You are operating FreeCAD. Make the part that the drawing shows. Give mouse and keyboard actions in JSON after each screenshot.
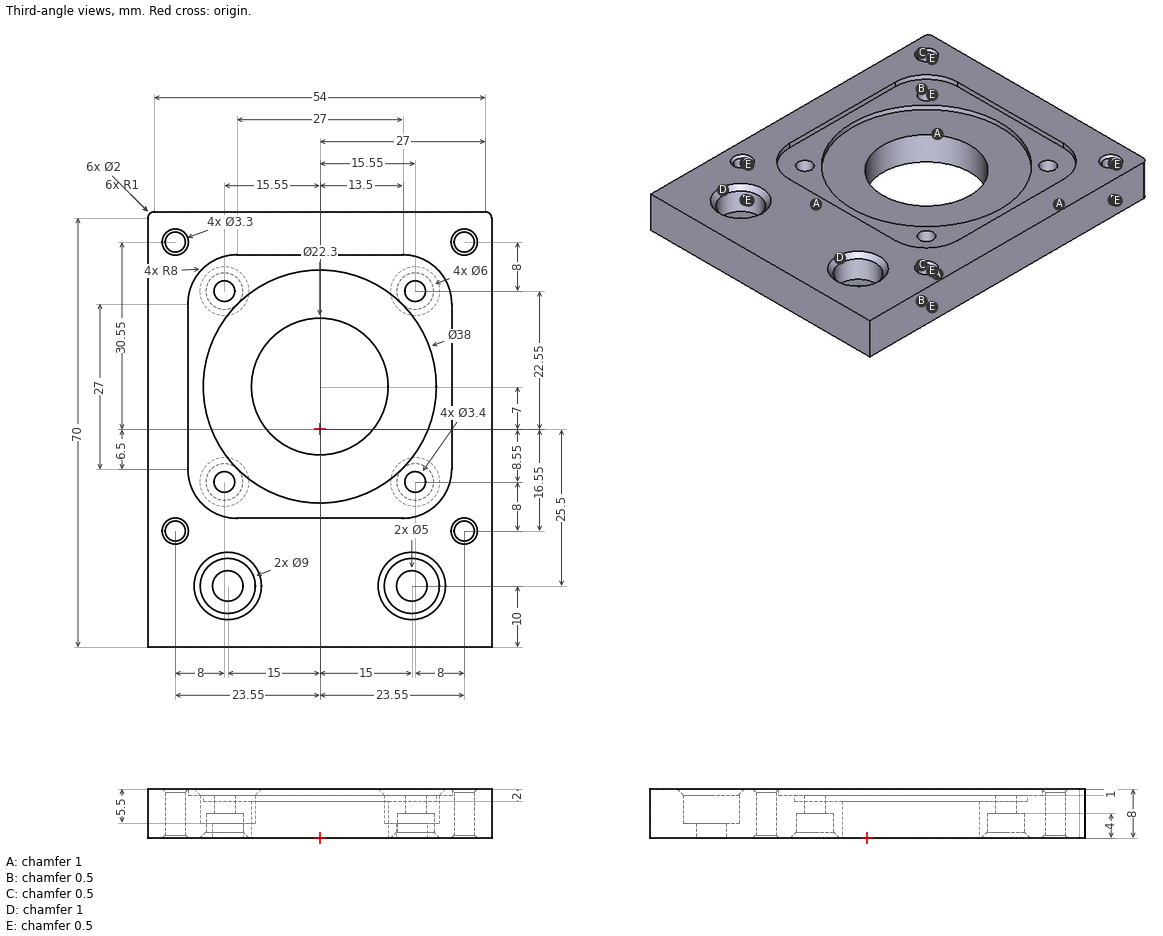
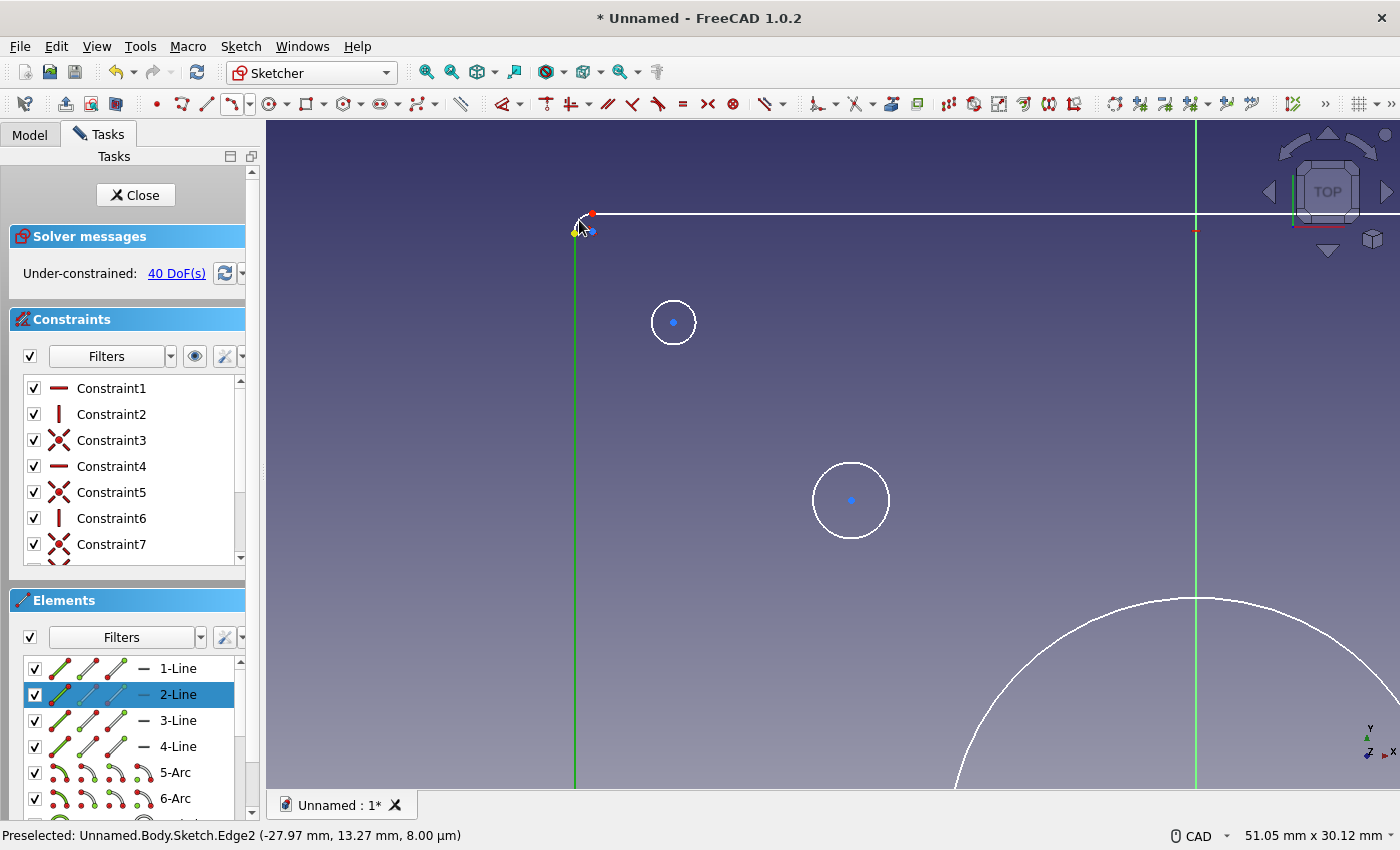
{"action": "left_click", "coordinate": [579, 220]}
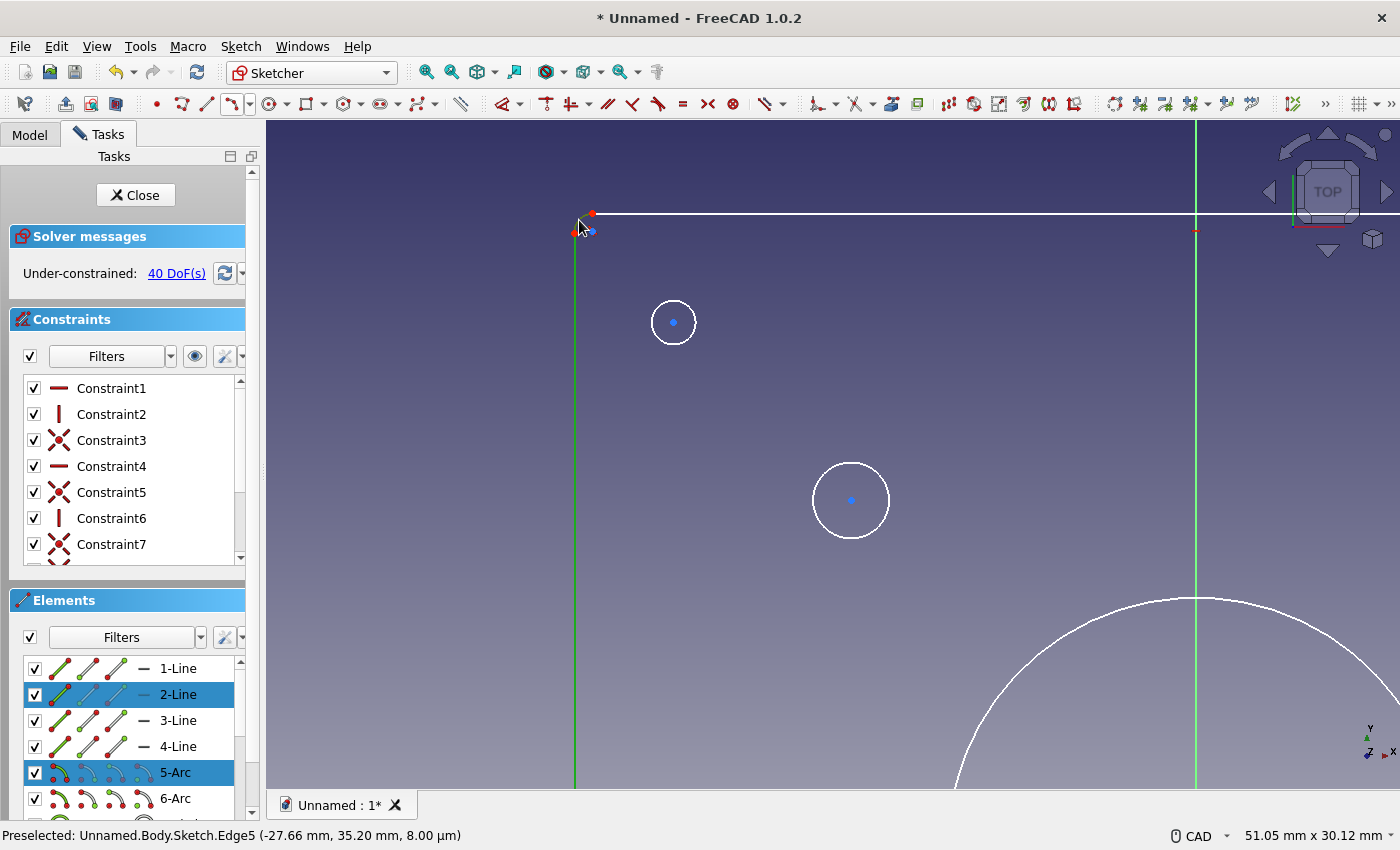
{"action": "key", "text": "t"}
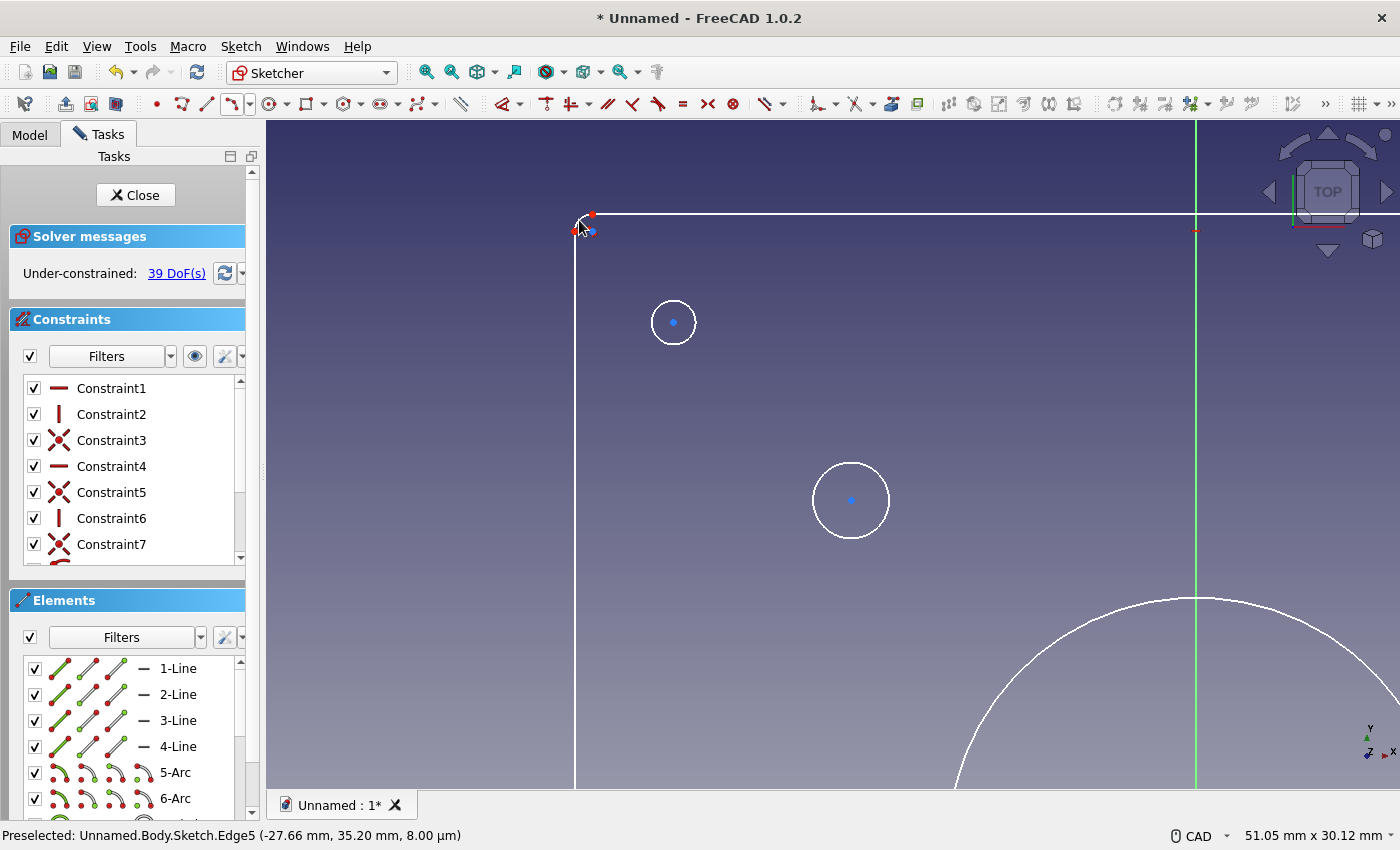
{"action": "scroll", "coordinate": [578, 220], "scroll_direction": "down", "scroll_amount": 6}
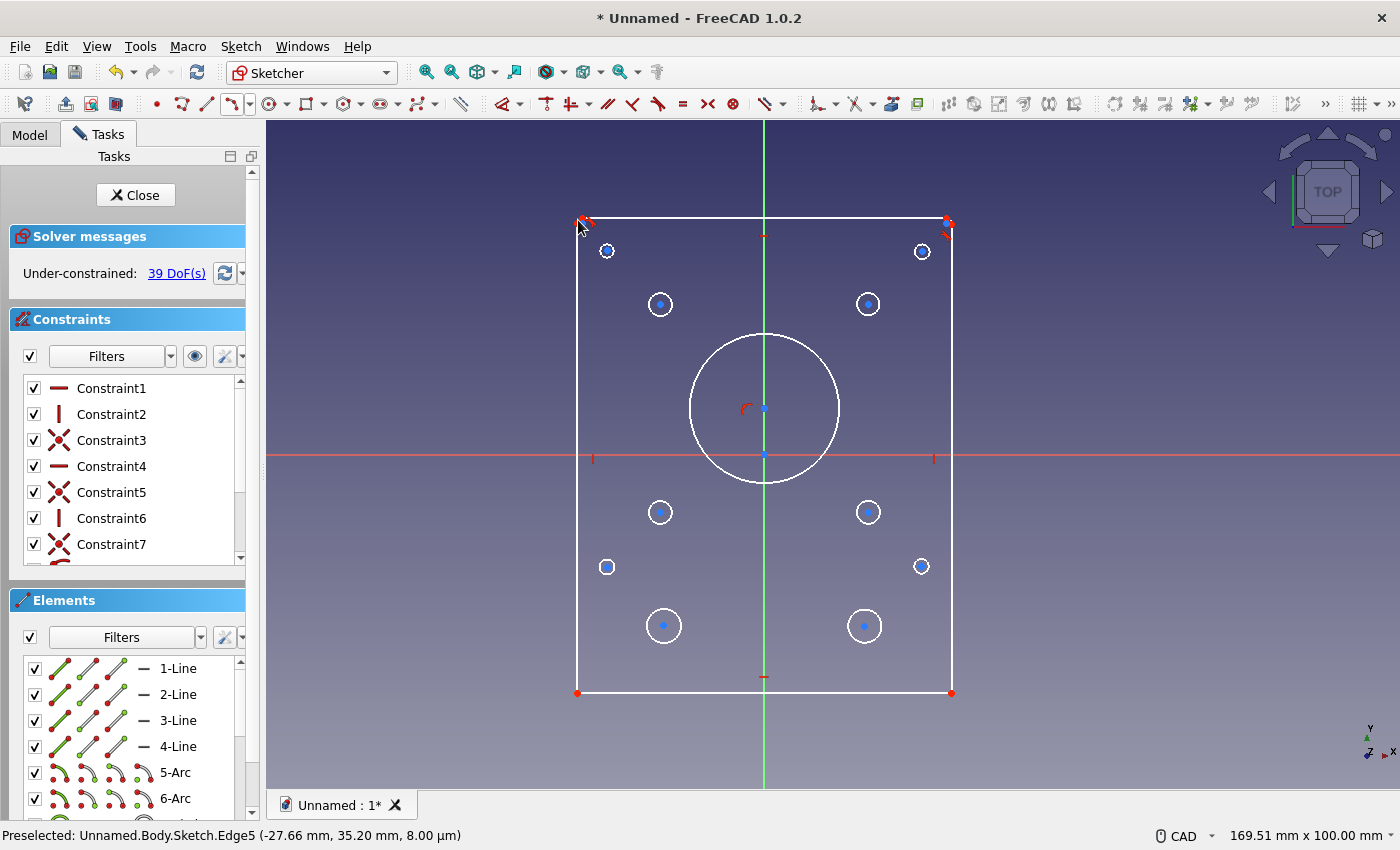
{"action": "left_click", "coordinate": [952, 553]}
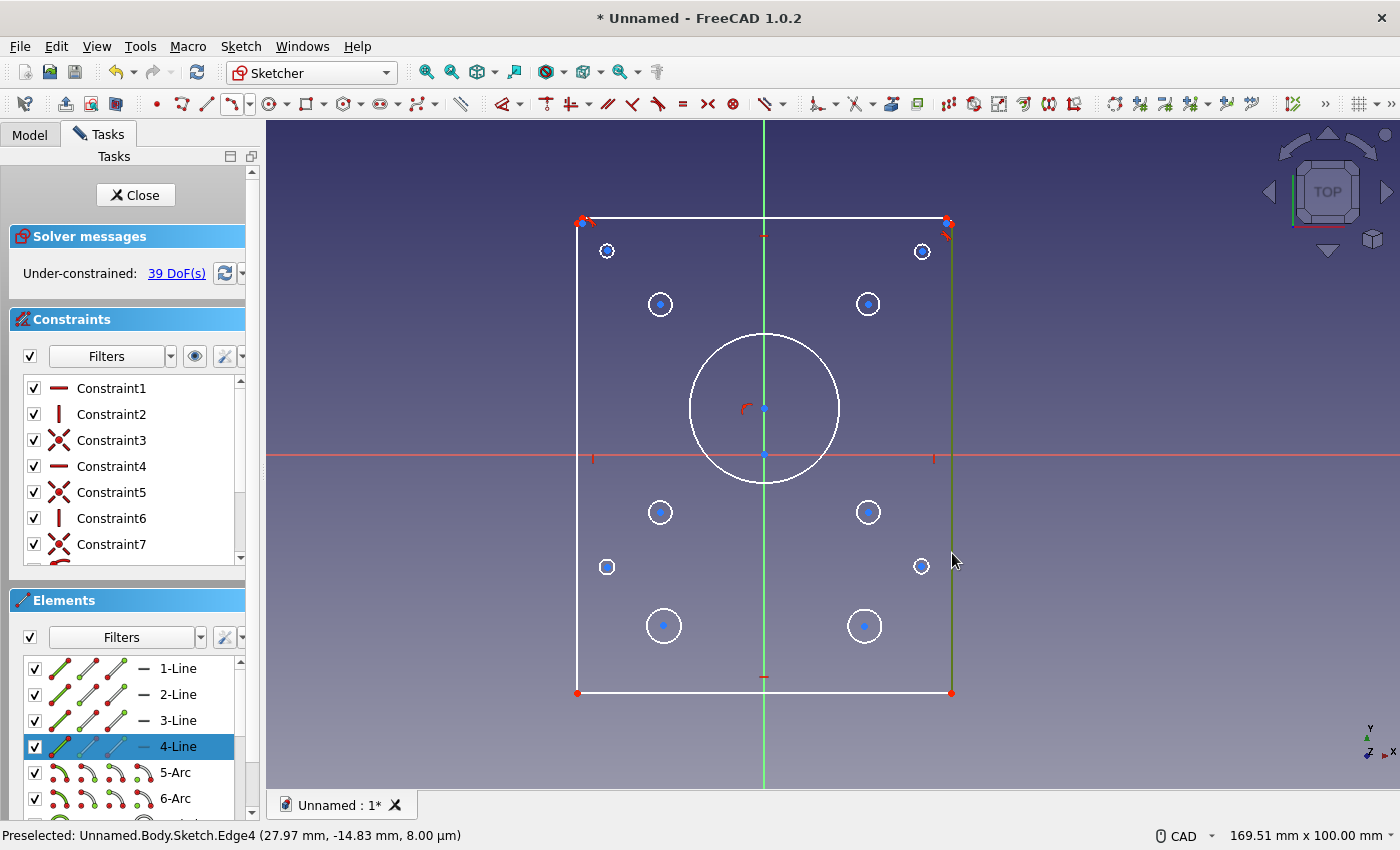
{"action": "scroll", "coordinate": [950, 220], "scroll_direction": "up", "scroll_amount": 6}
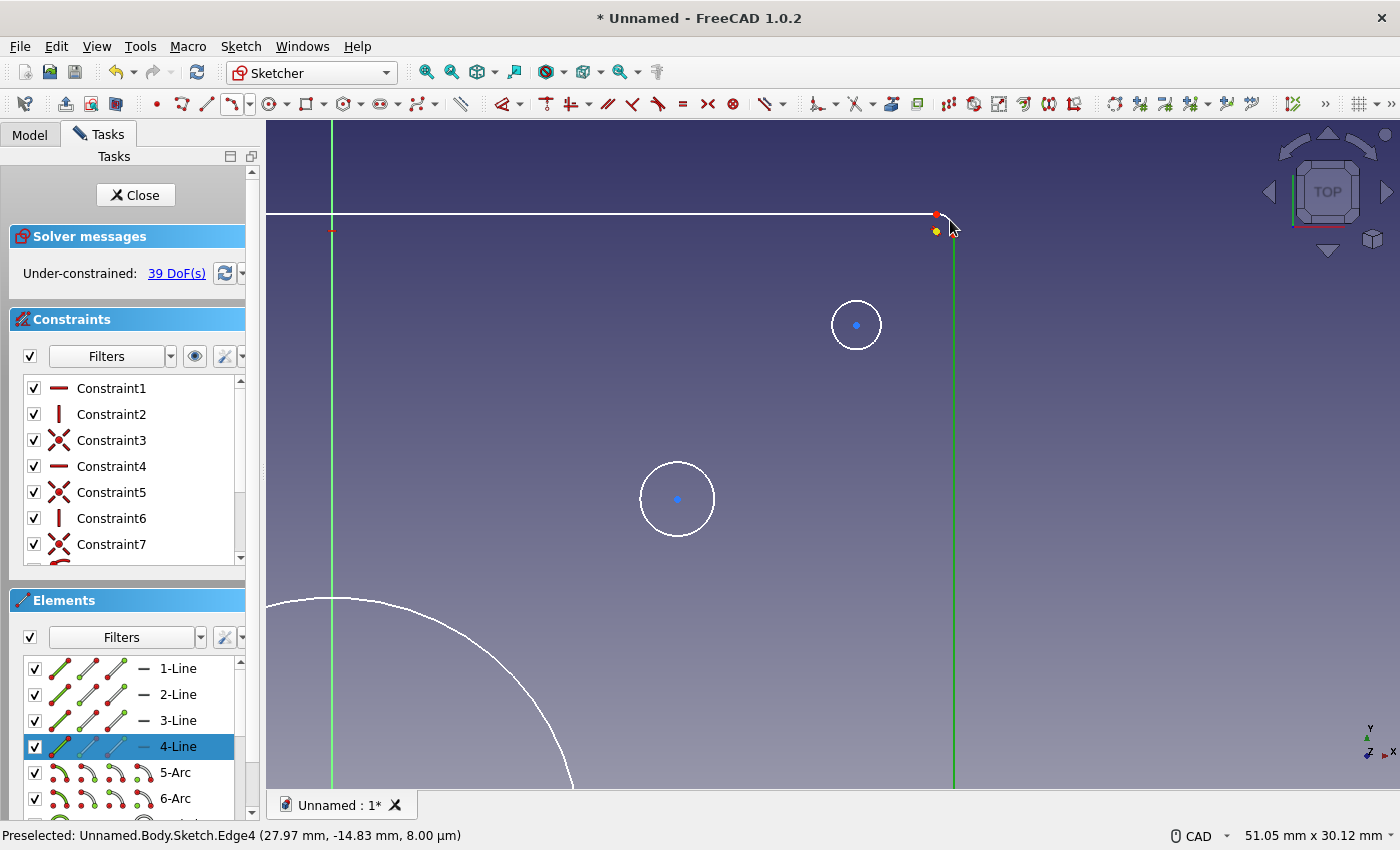
{"action": "left_click", "coordinate": [950, 220]}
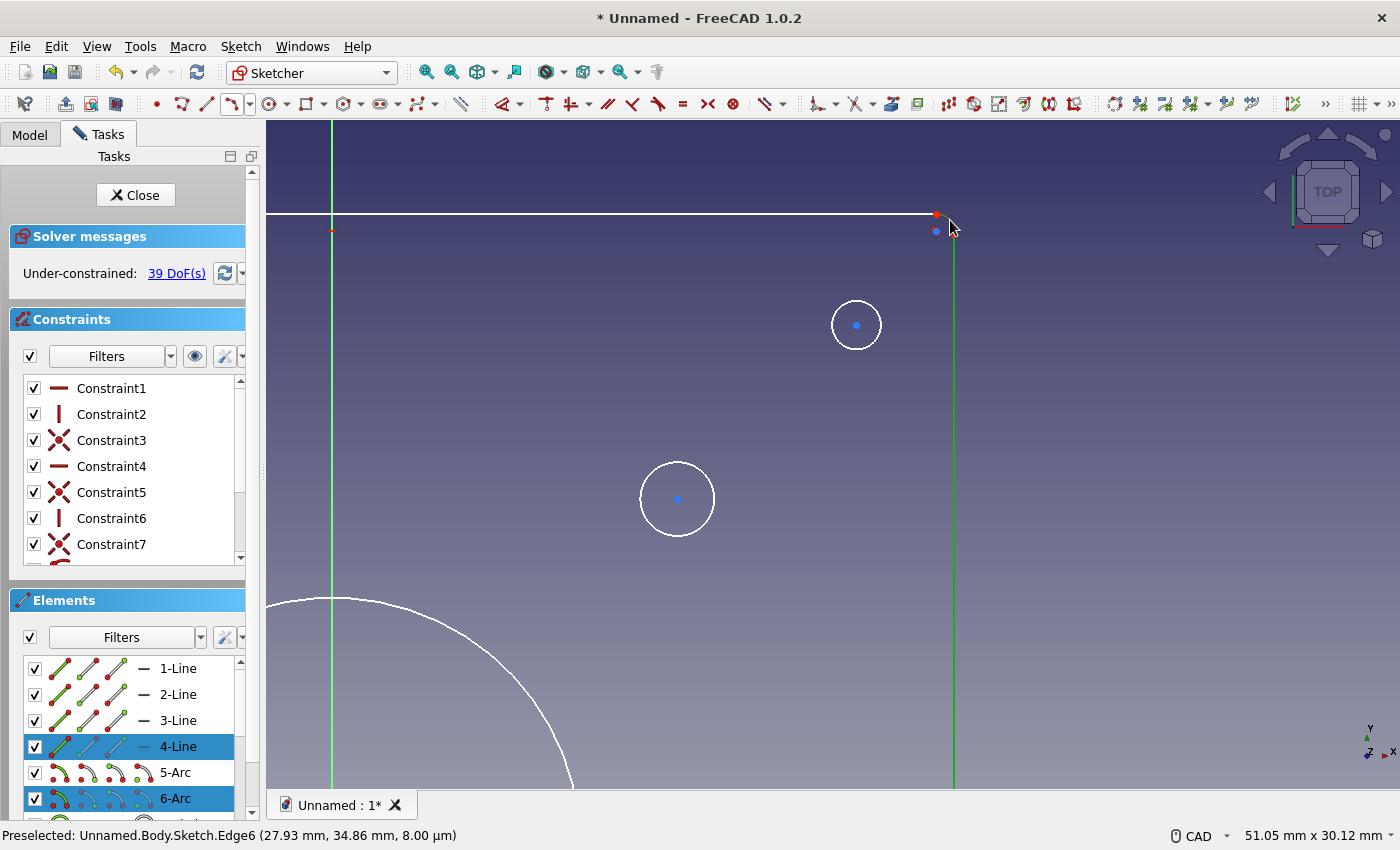
{"action": "key", "text": "t"}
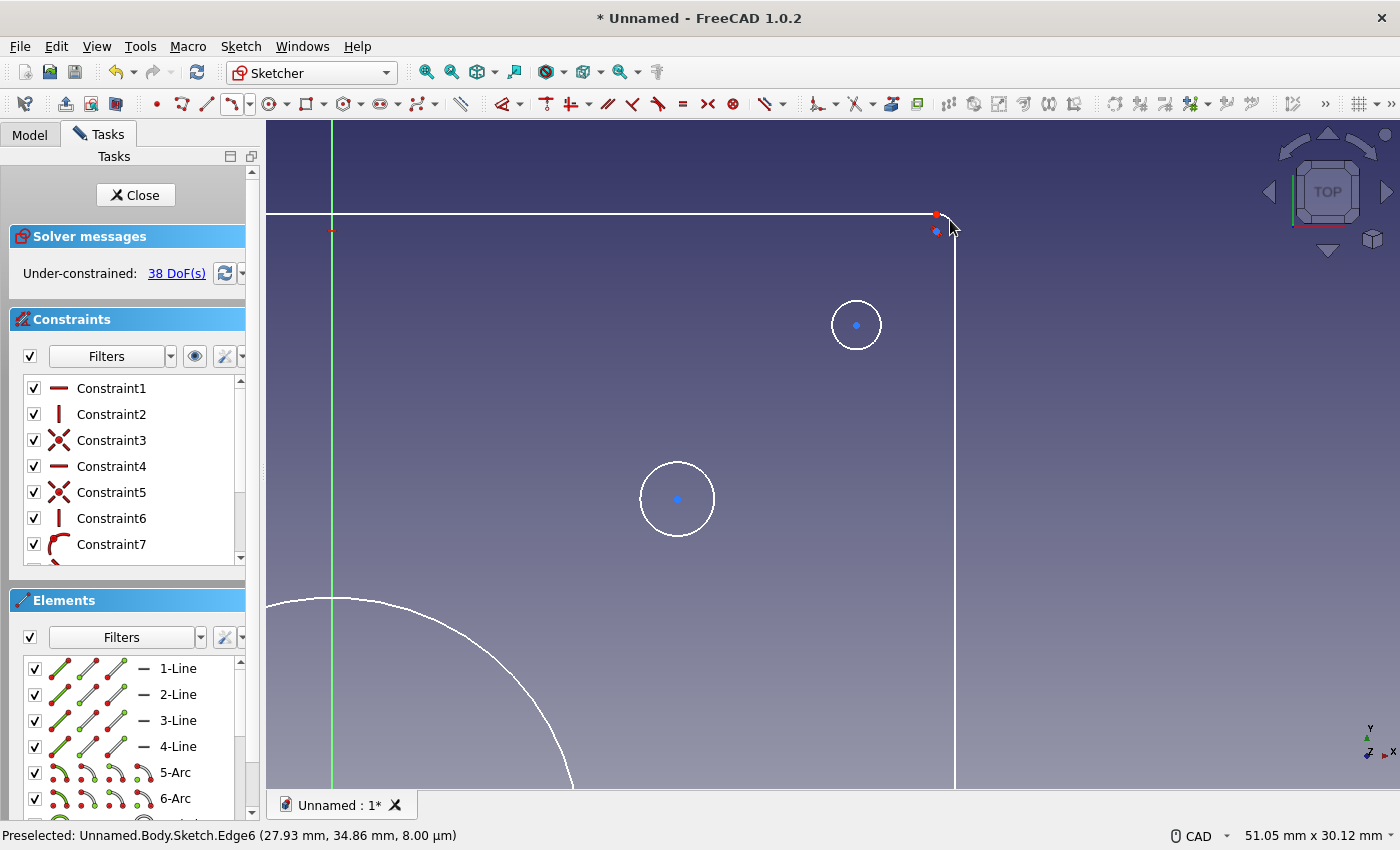
{"action": "scroll", "coordinate": [951, 220], "scroll_direction": "down", "scroll_amount": 6}